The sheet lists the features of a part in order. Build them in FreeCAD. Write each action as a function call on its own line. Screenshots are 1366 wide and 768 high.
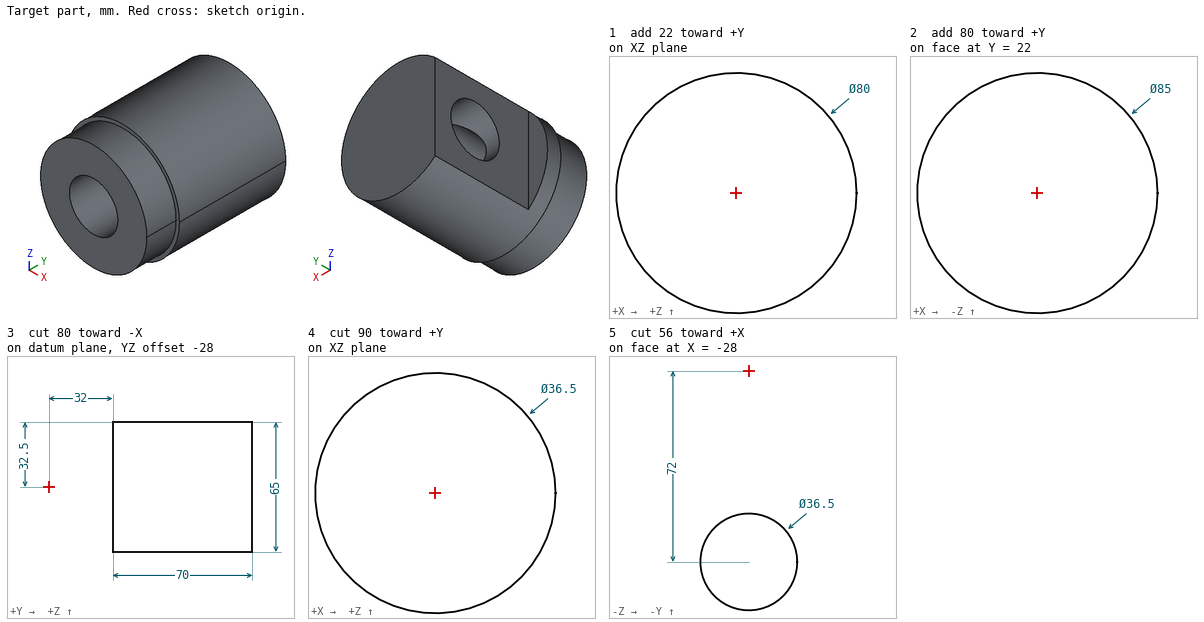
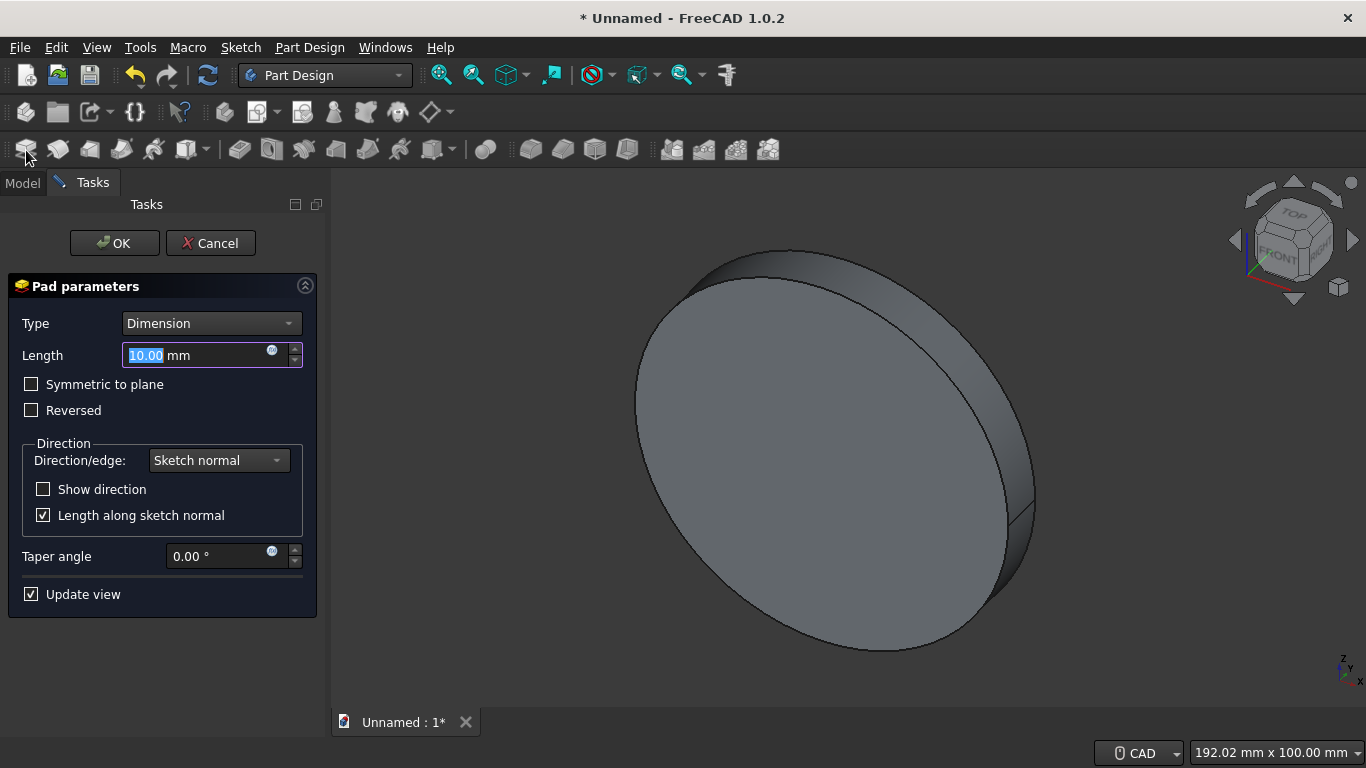
text(22)
key(Tab)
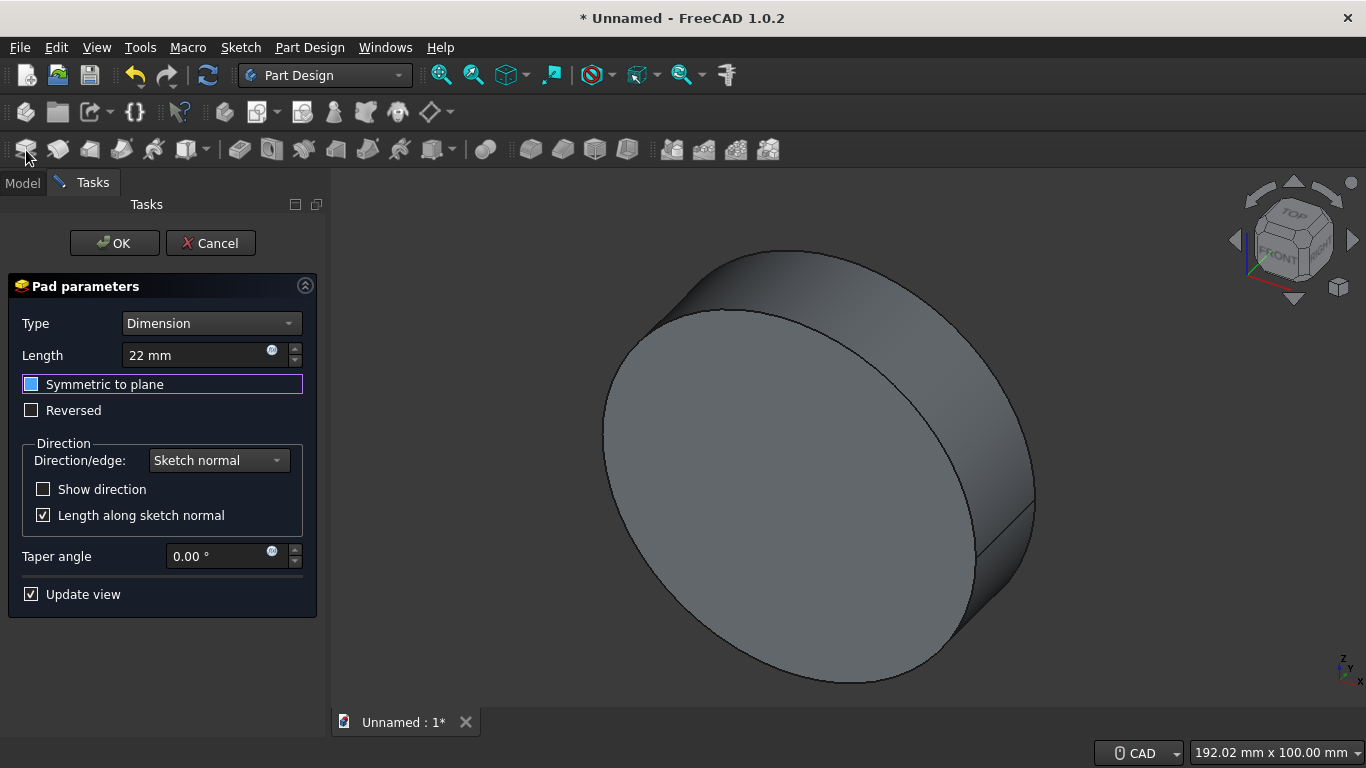
click(30, 410)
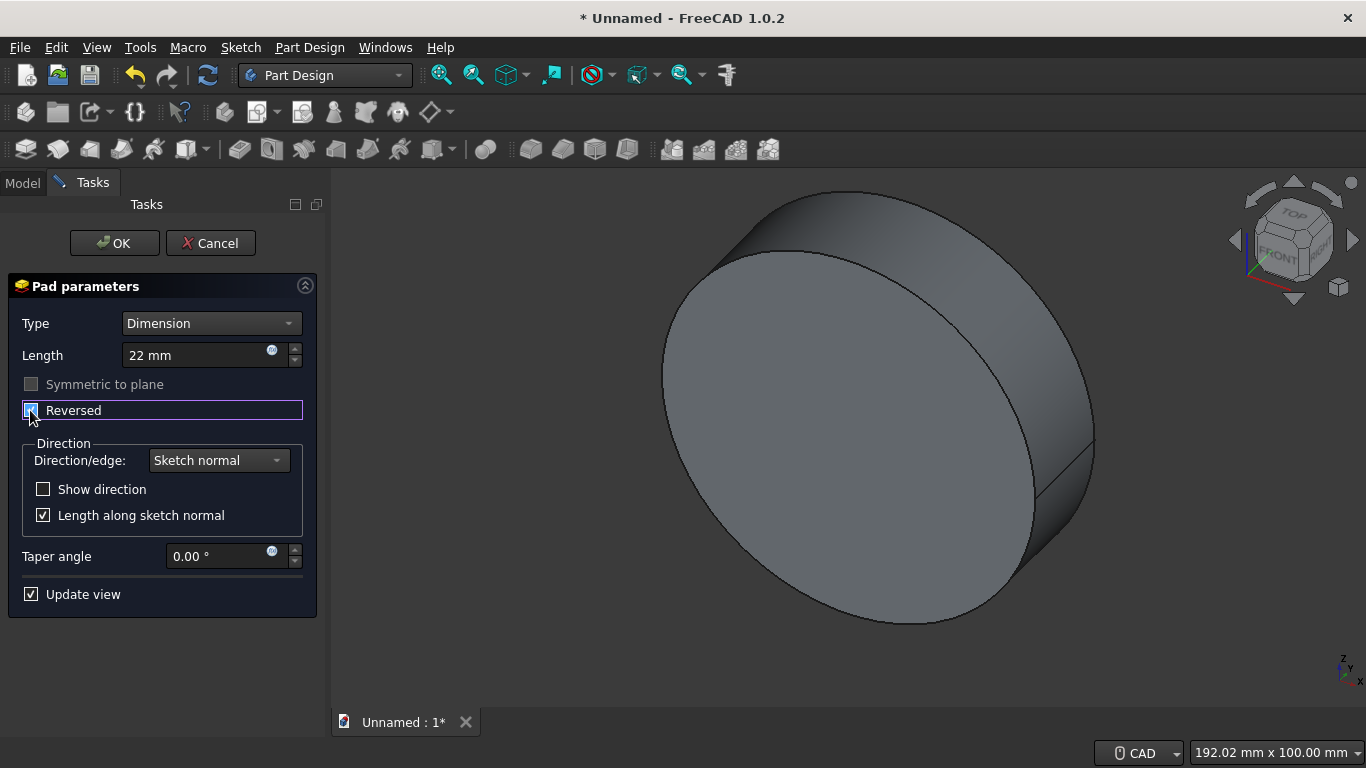
click(115, 243)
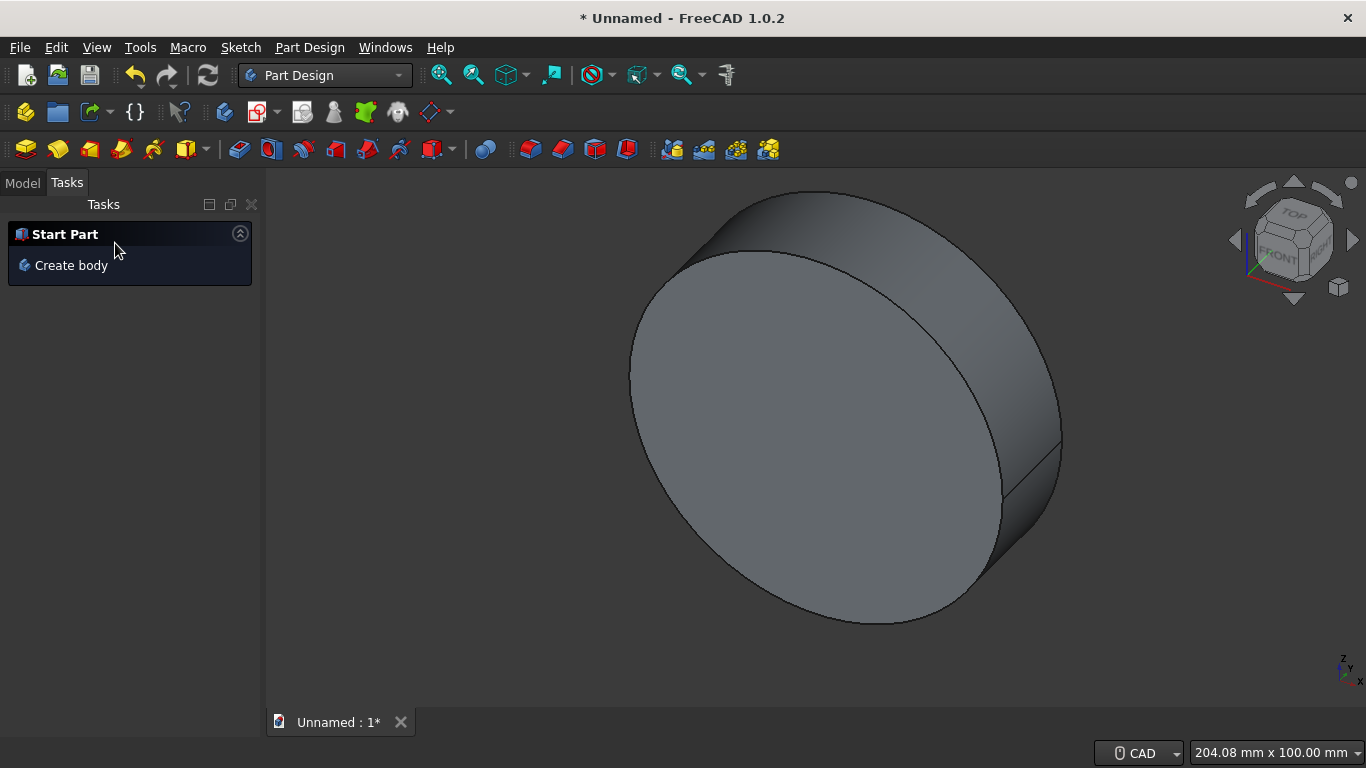
click(442, 76)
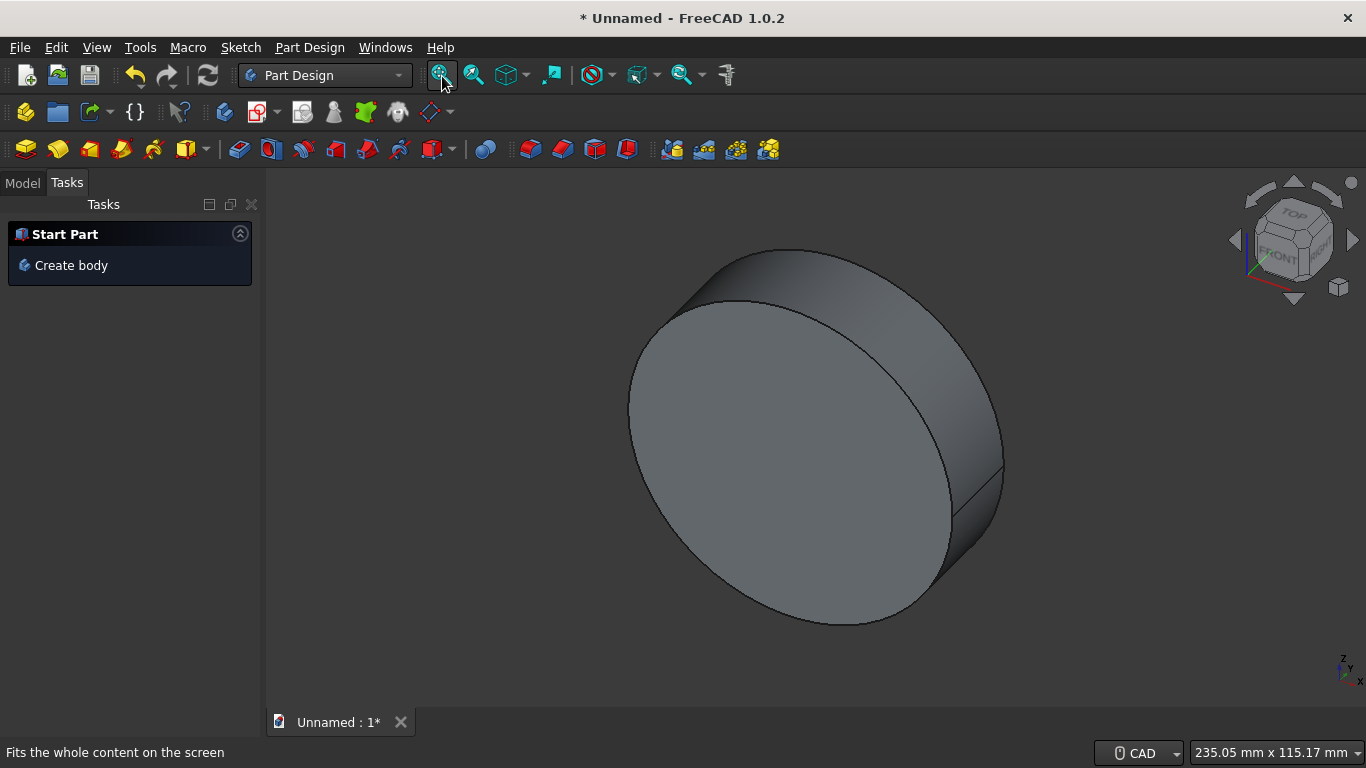
key(4)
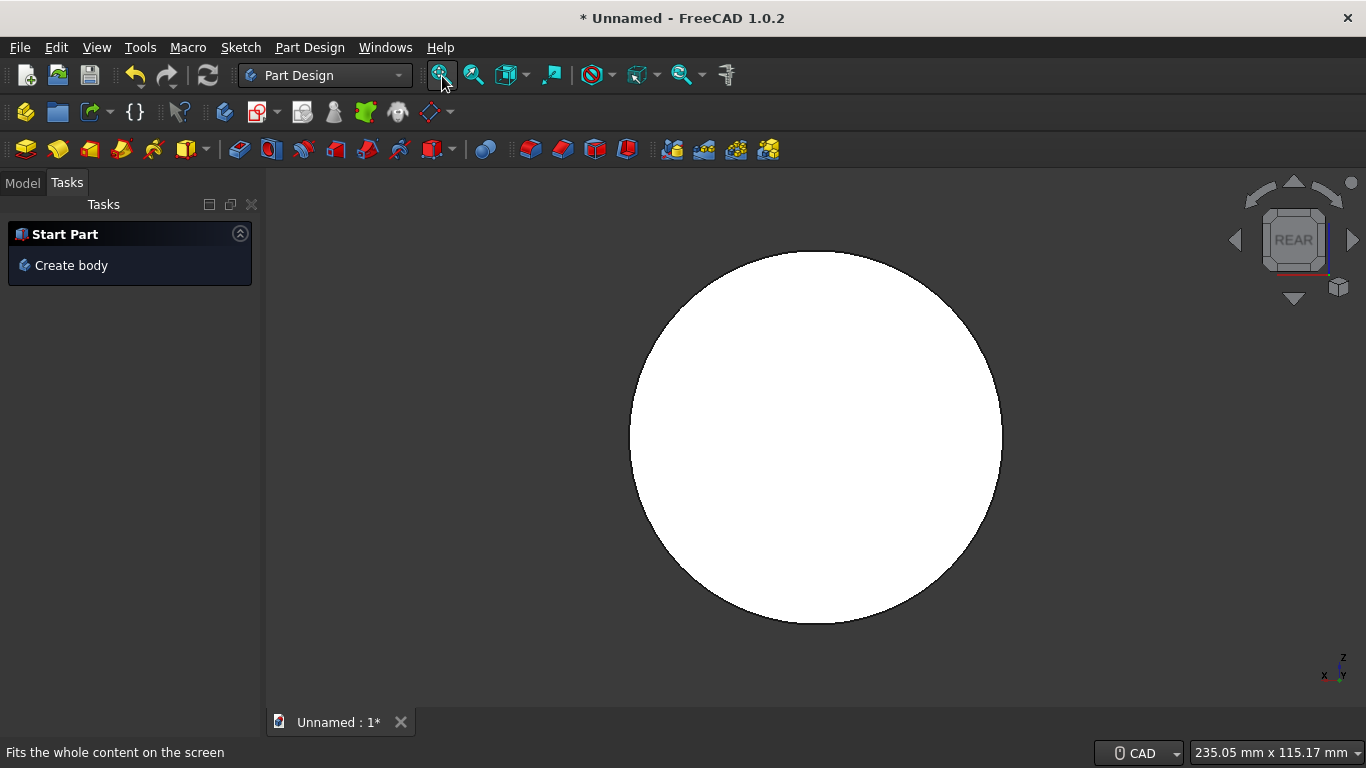
click(816, 437)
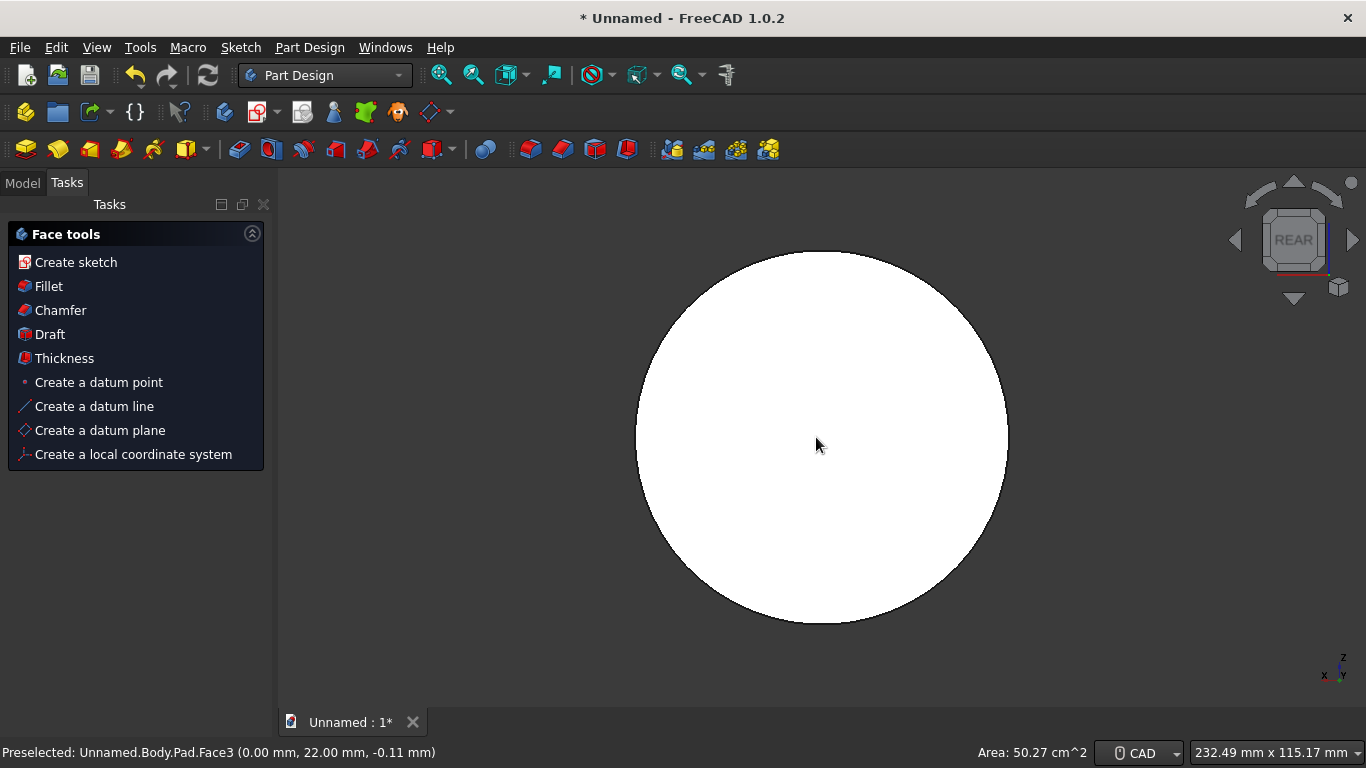
click(258, 112)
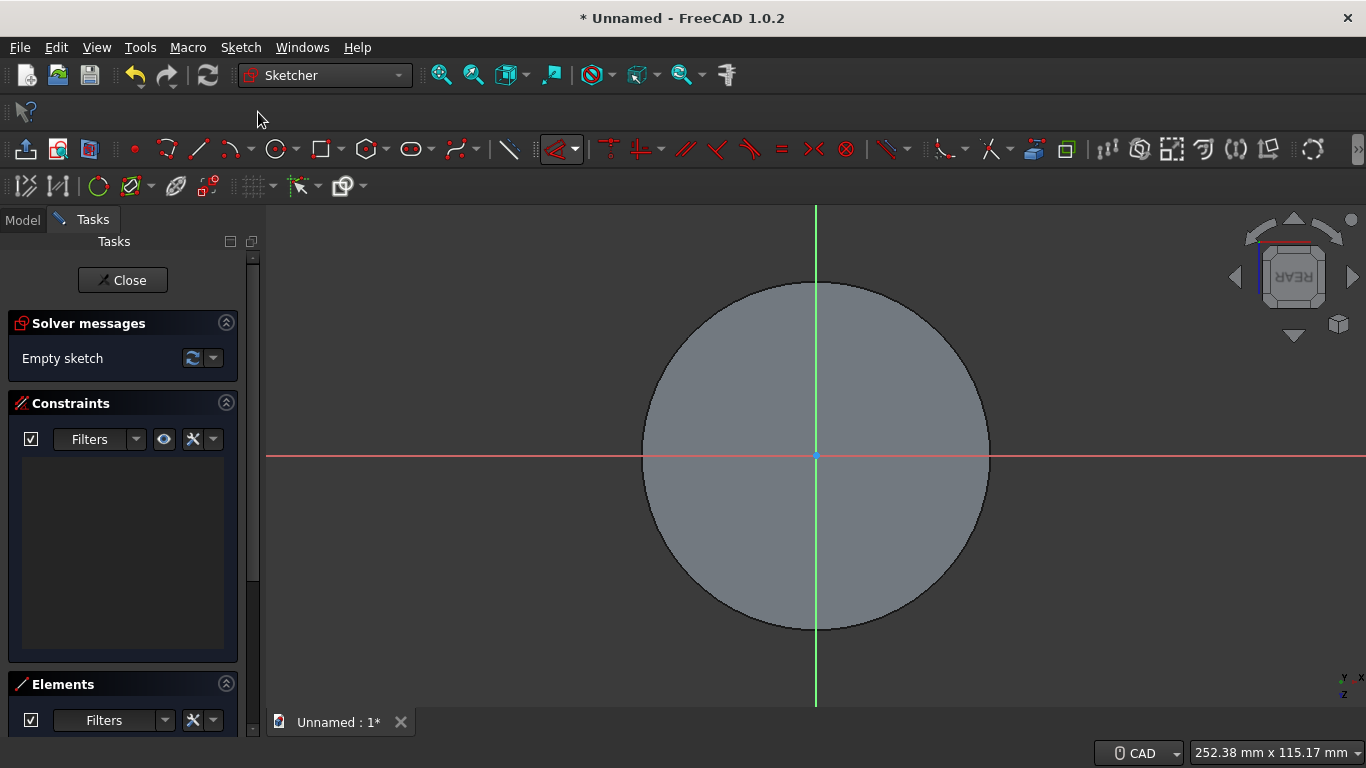
click(276, 150)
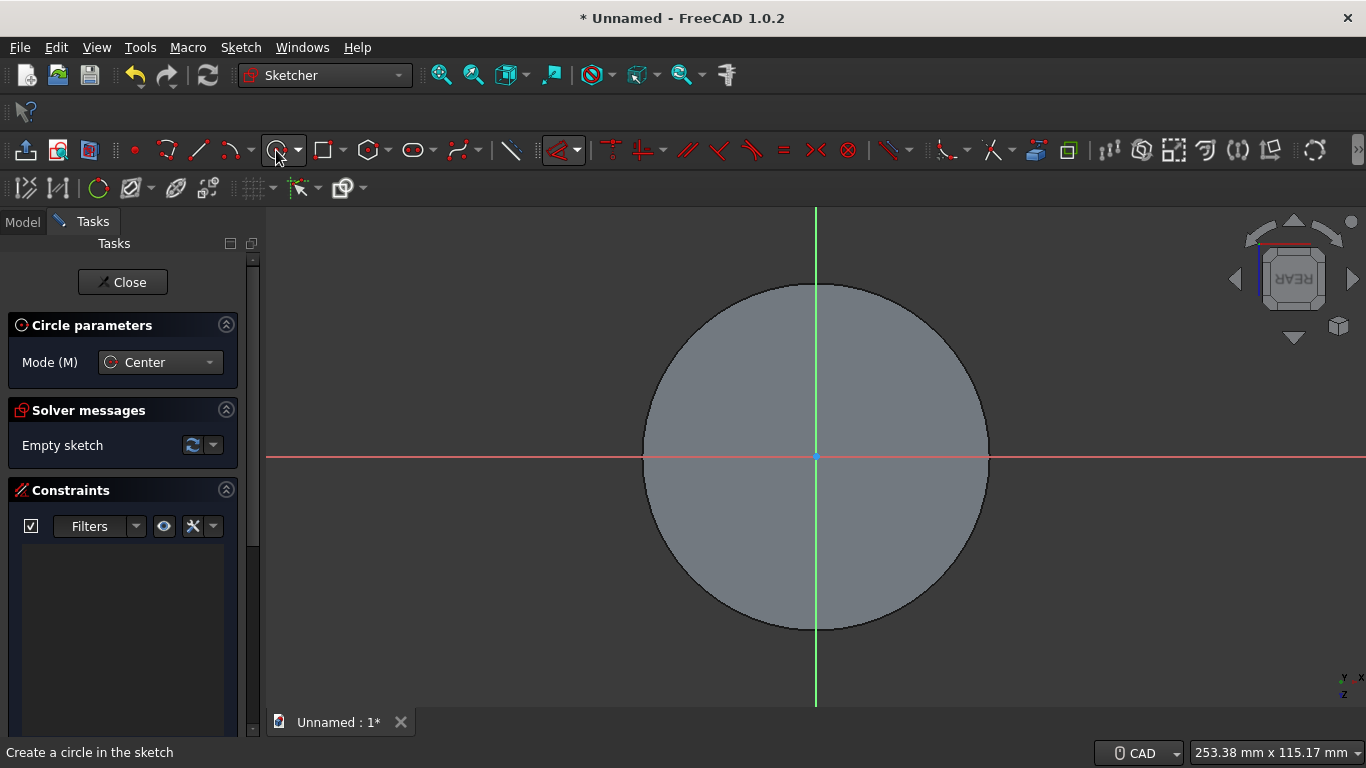
click(816, 457)
move(946, 327)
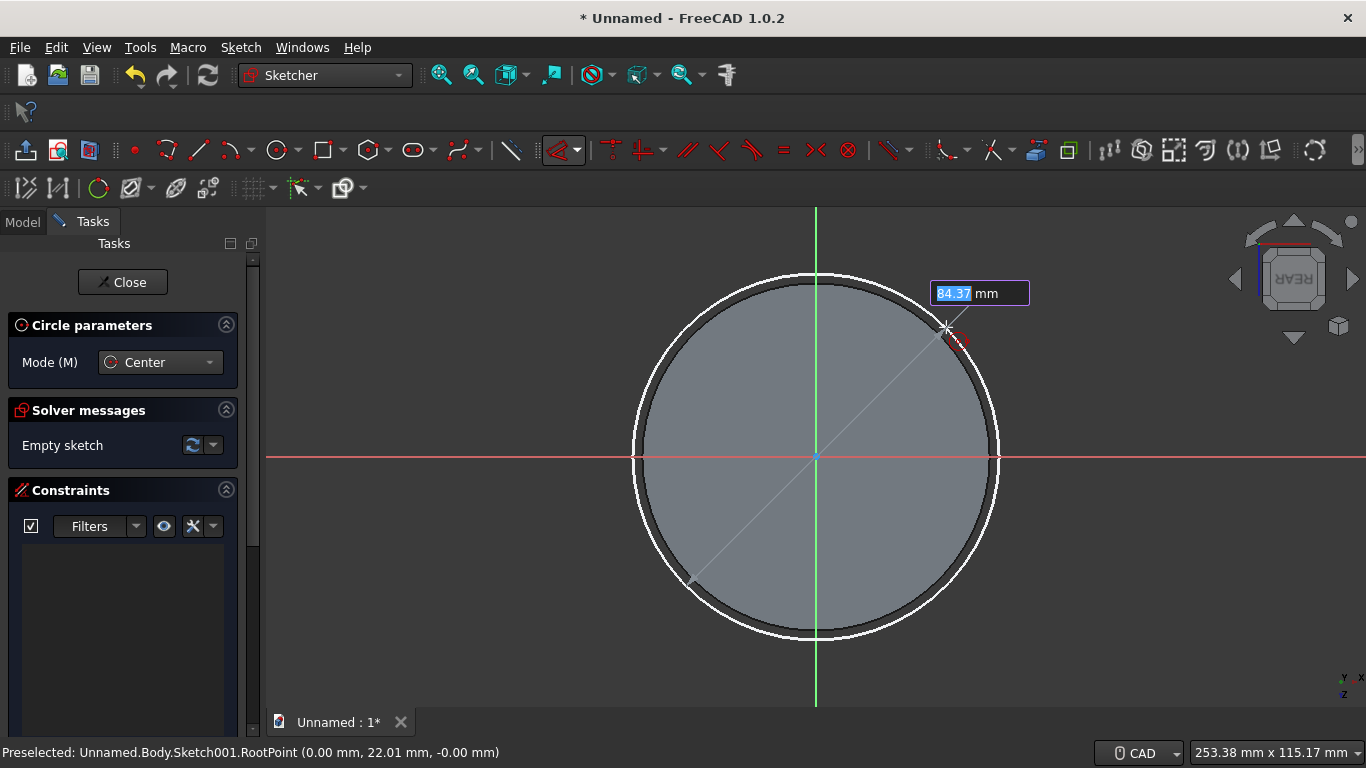
text(85)
key(Return)
key(Escape)